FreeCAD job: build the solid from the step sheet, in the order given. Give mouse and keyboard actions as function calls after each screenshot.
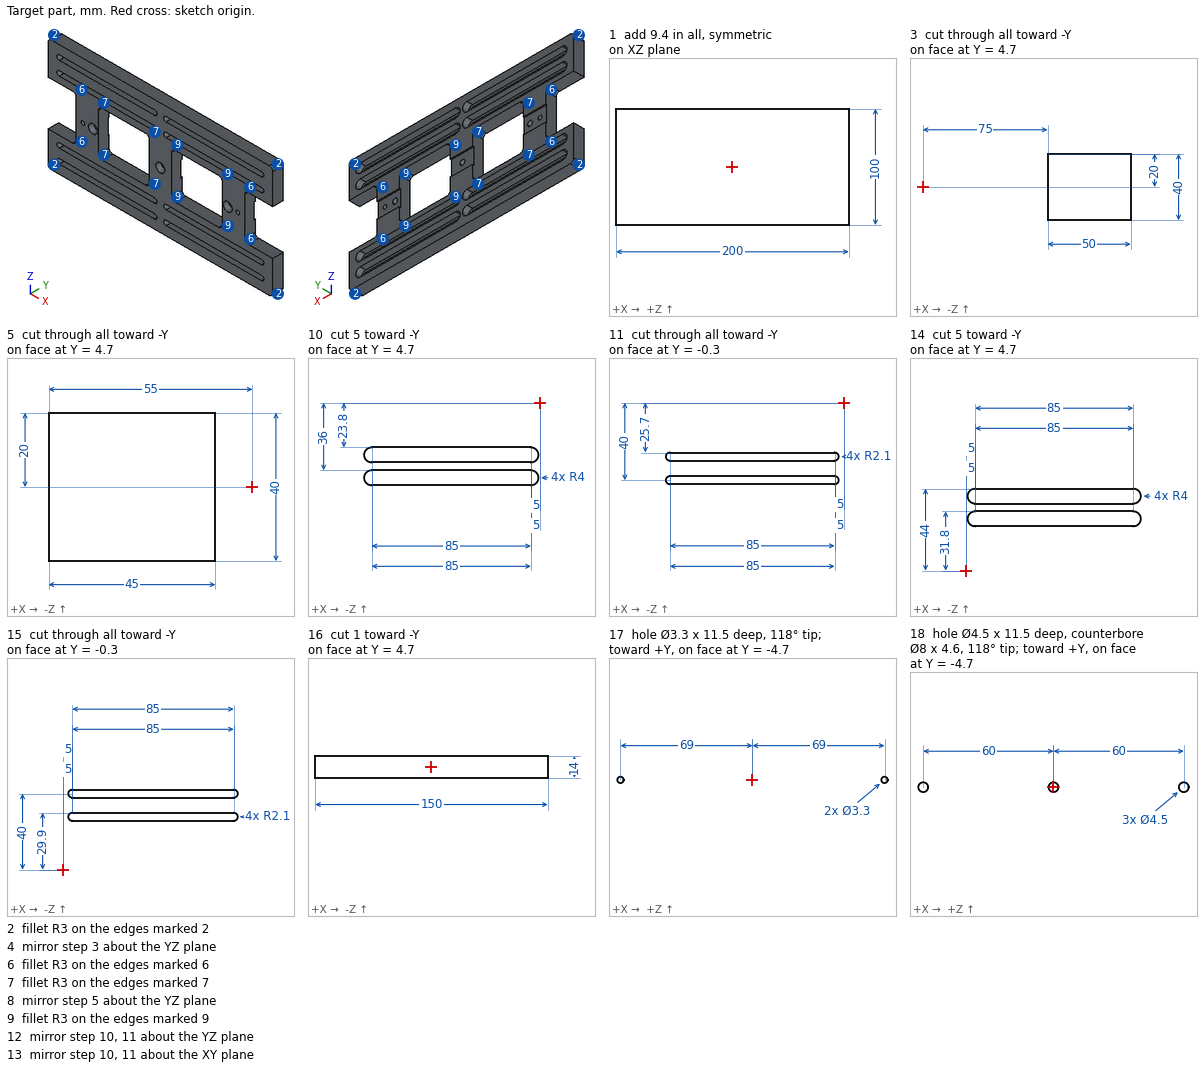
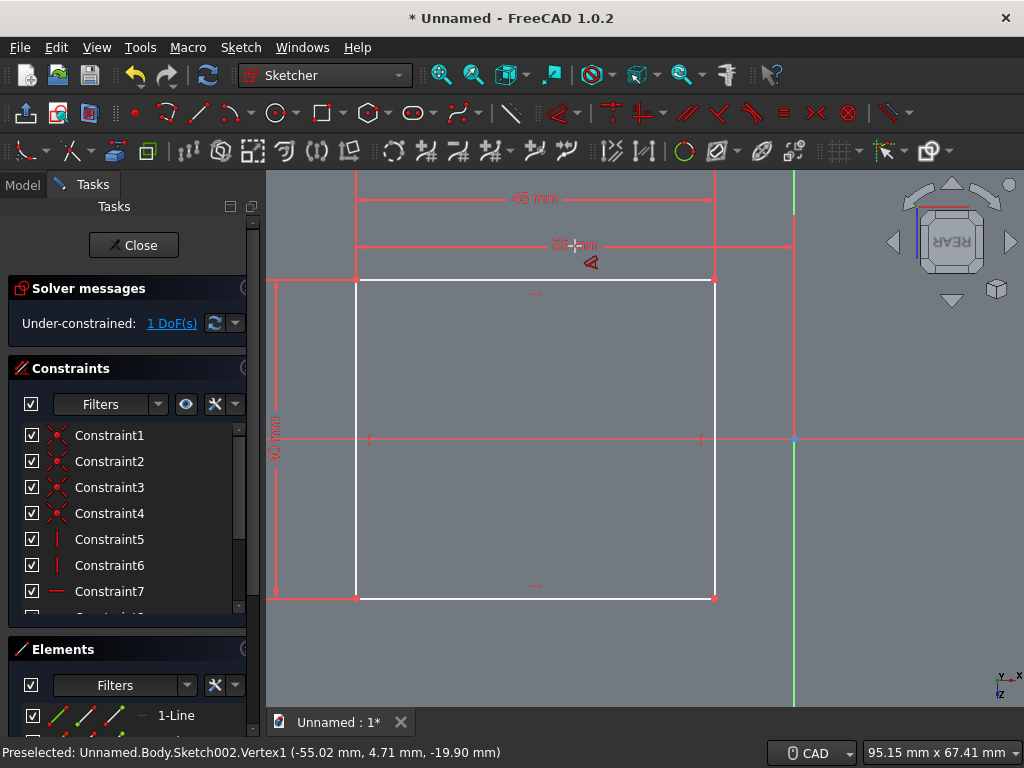
click(356, 280)
click(828, 359)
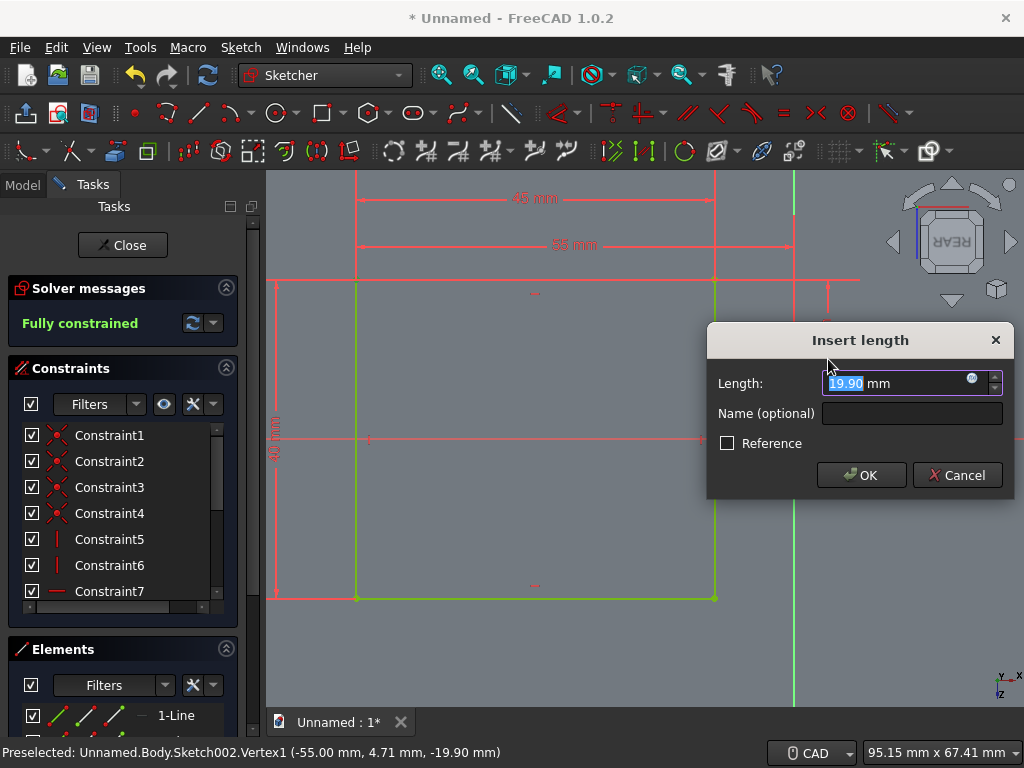
text(20)
key(Return)
key(Escape)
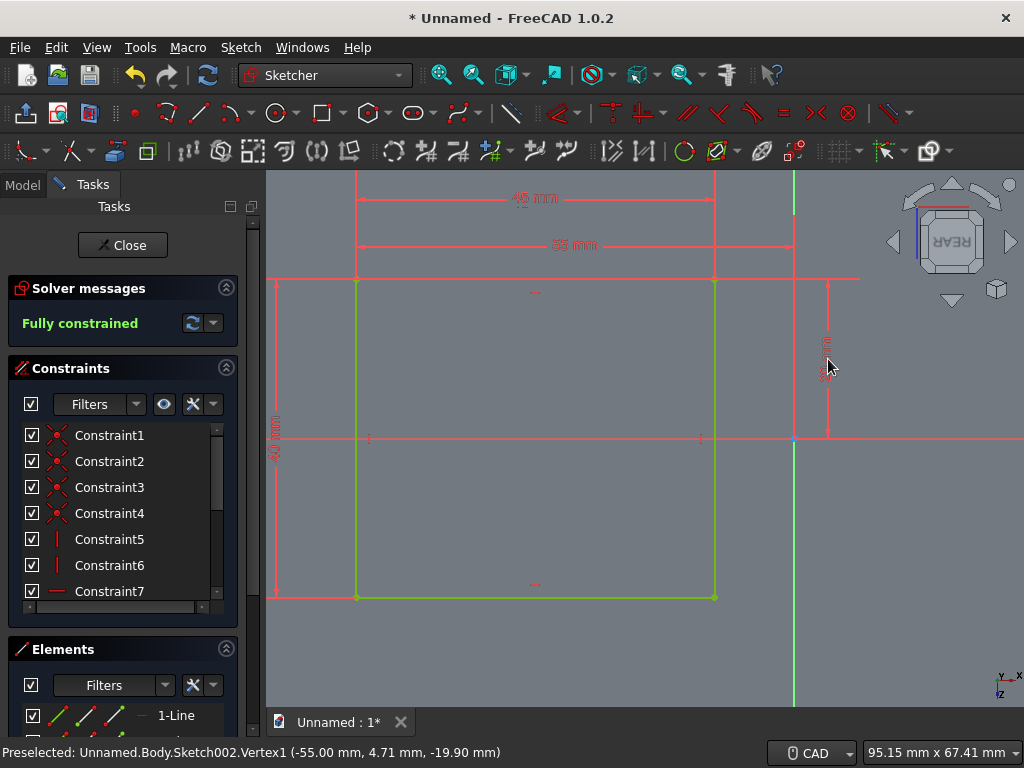
click(123, 245)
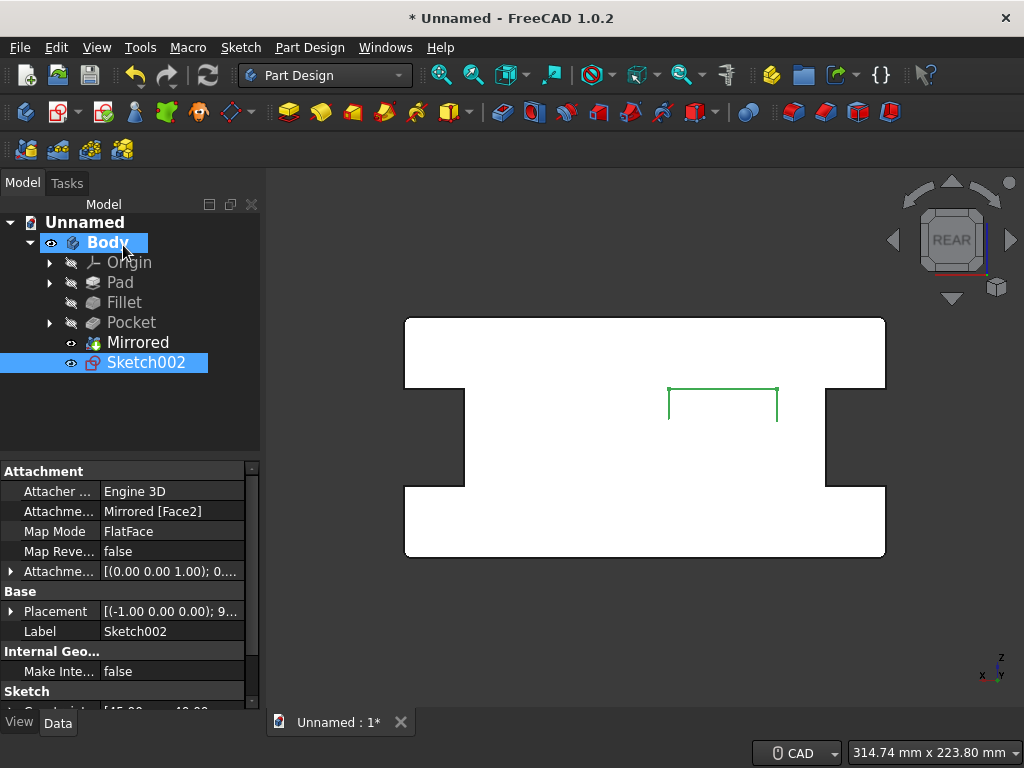
click(504, 112)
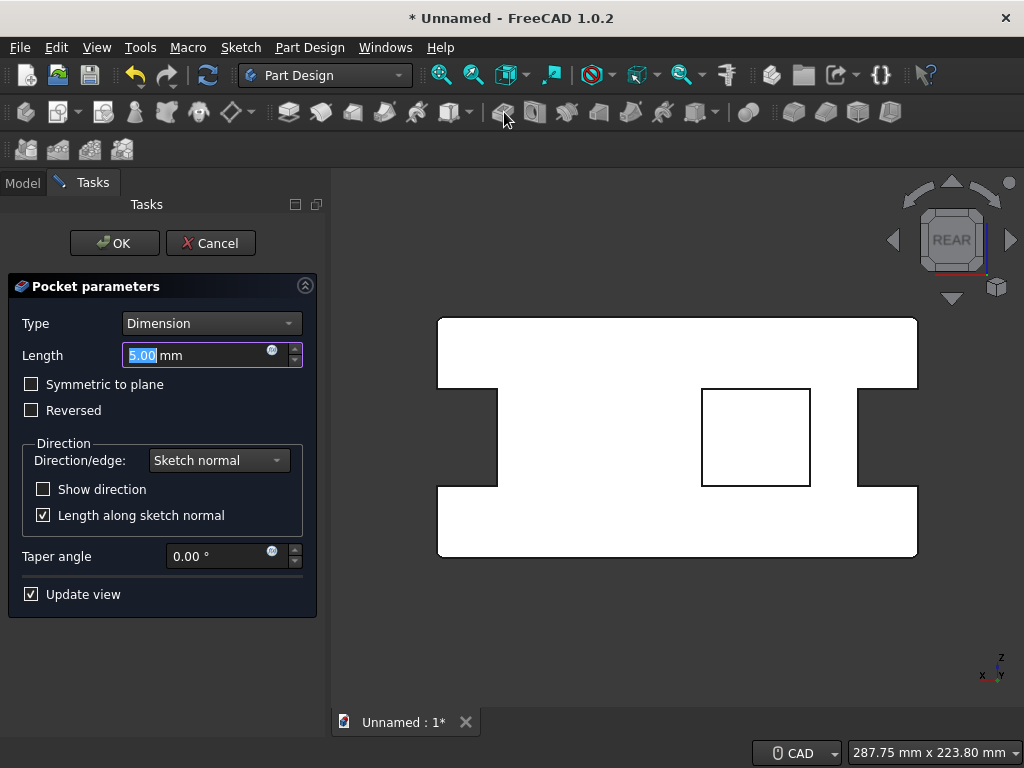
click(212, 324)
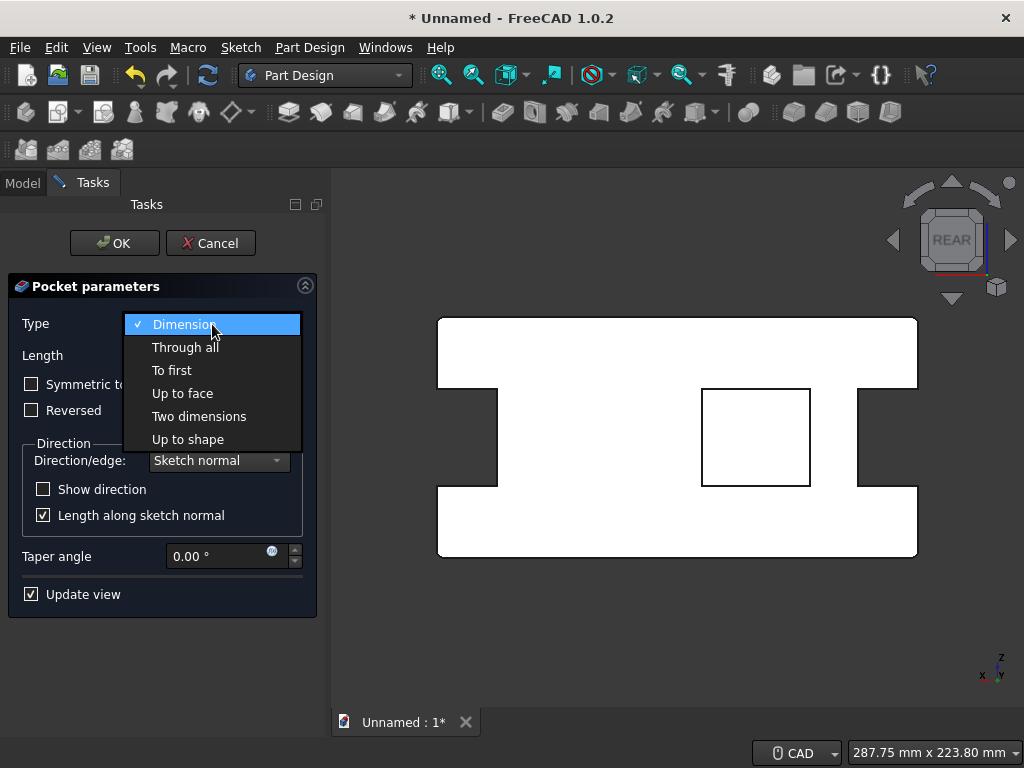
click(212, 348)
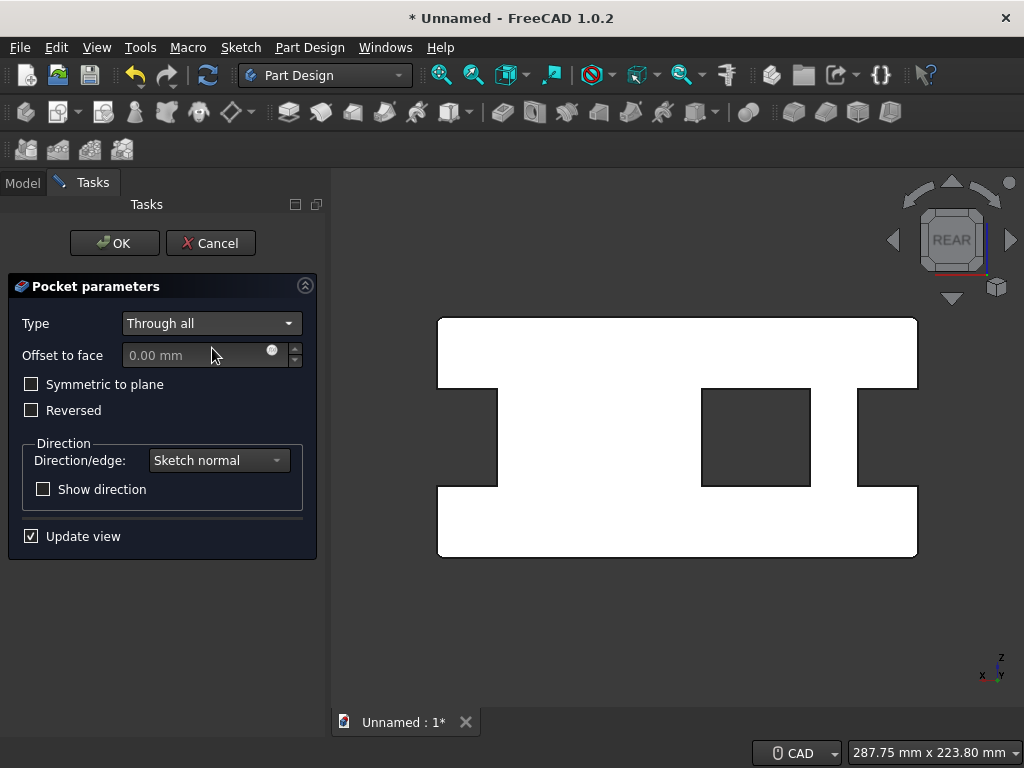
click(115, 243)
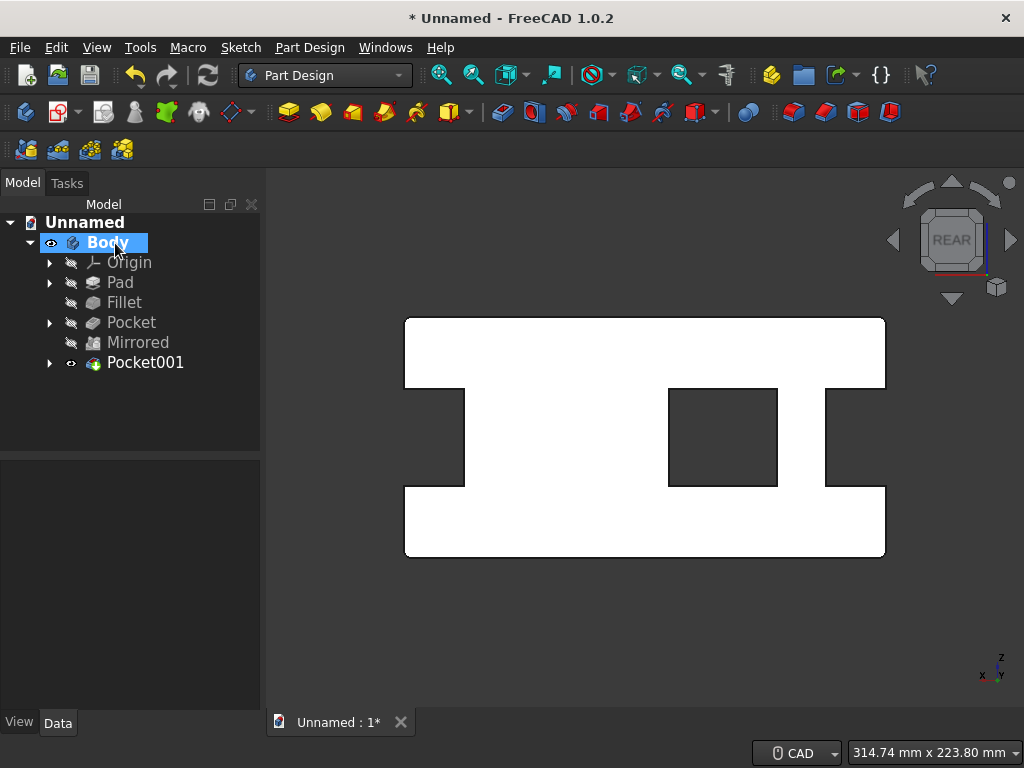
key(0)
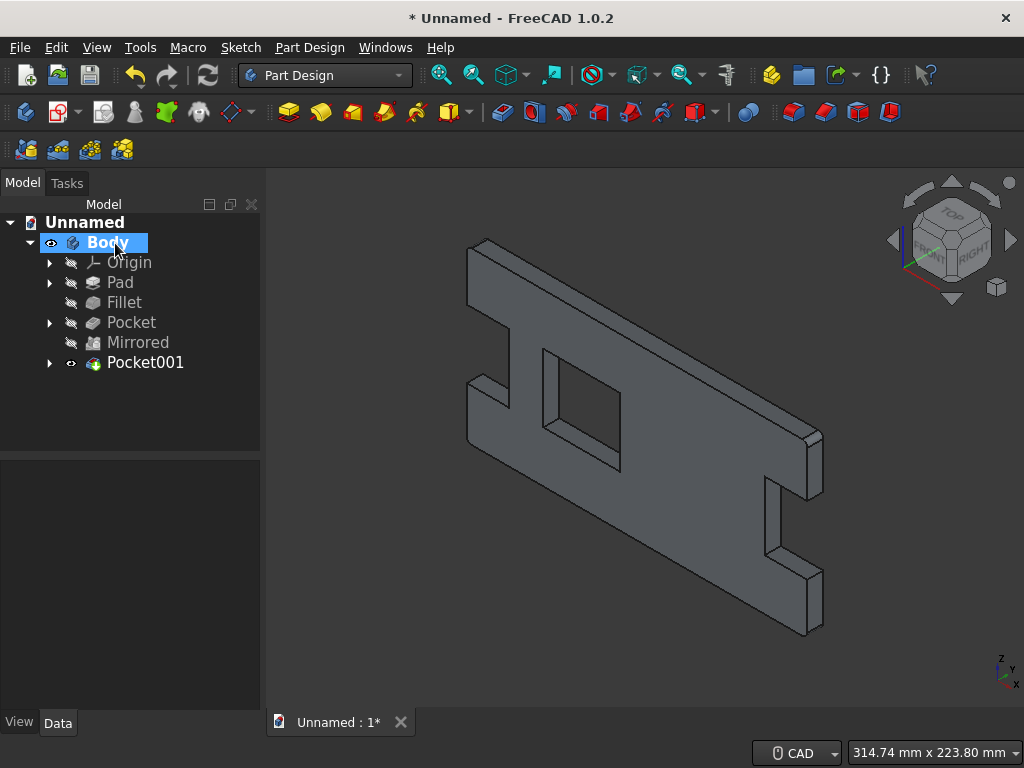
key(2)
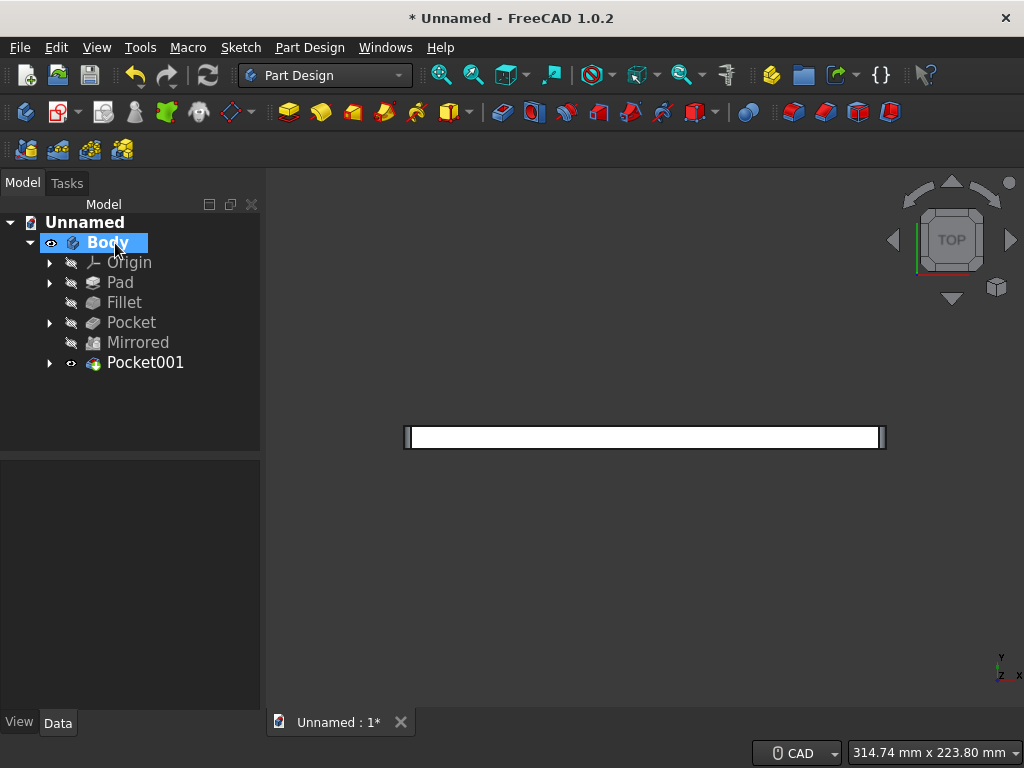
key(1)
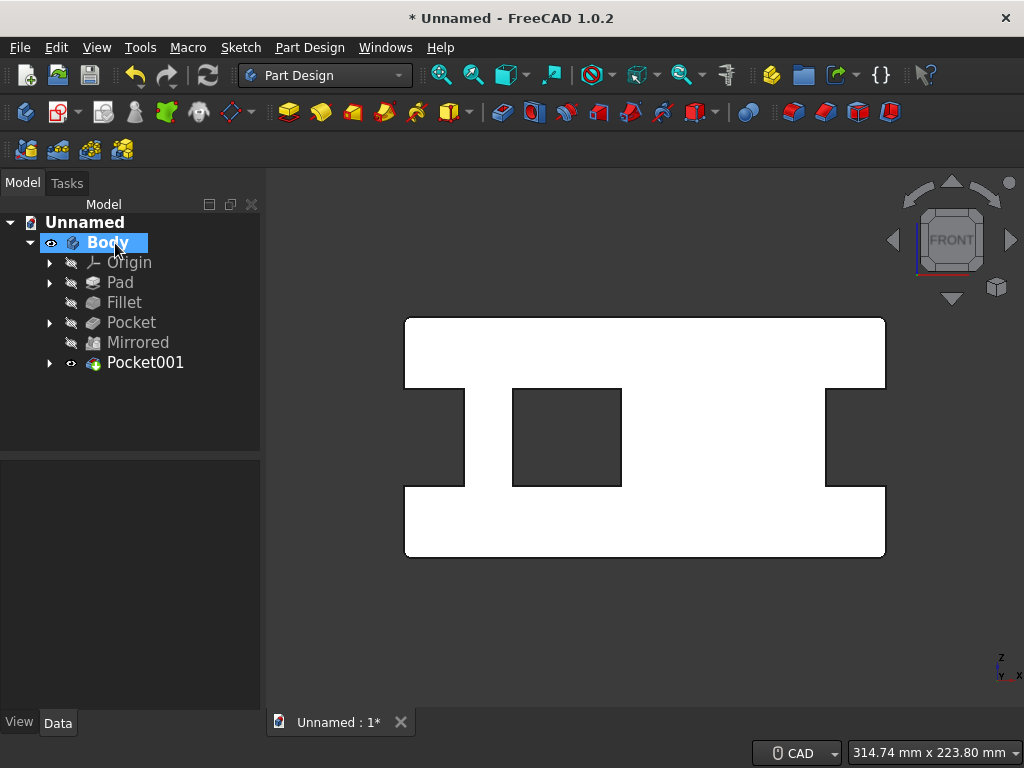
key(3)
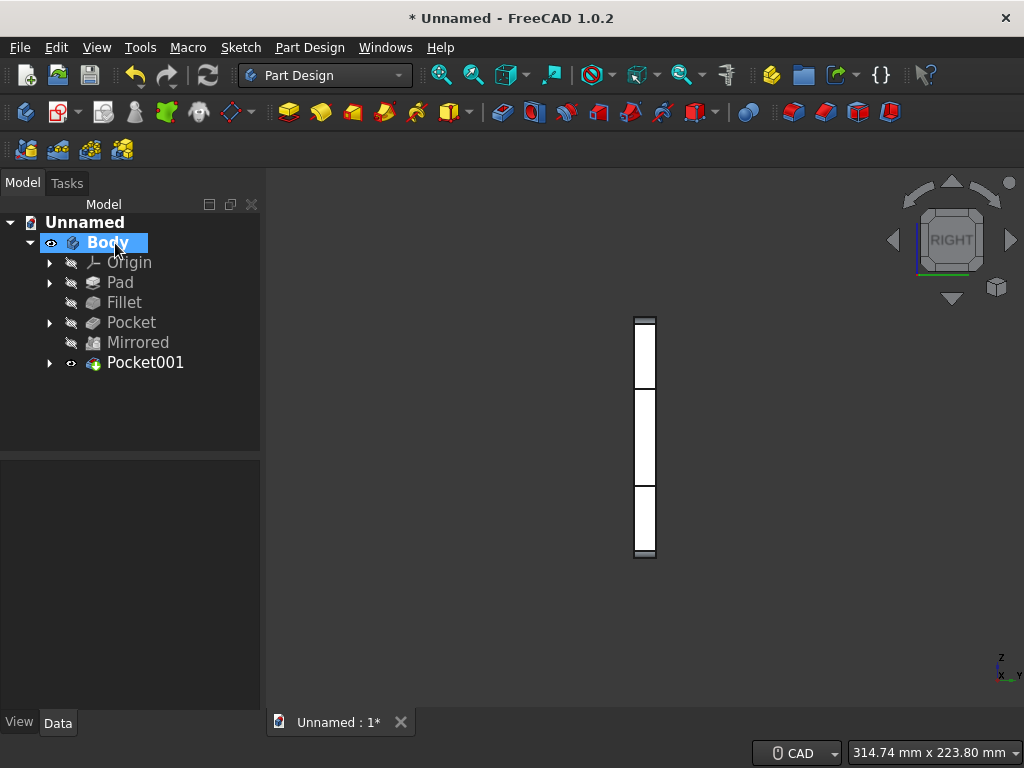
key(v)
key(f)